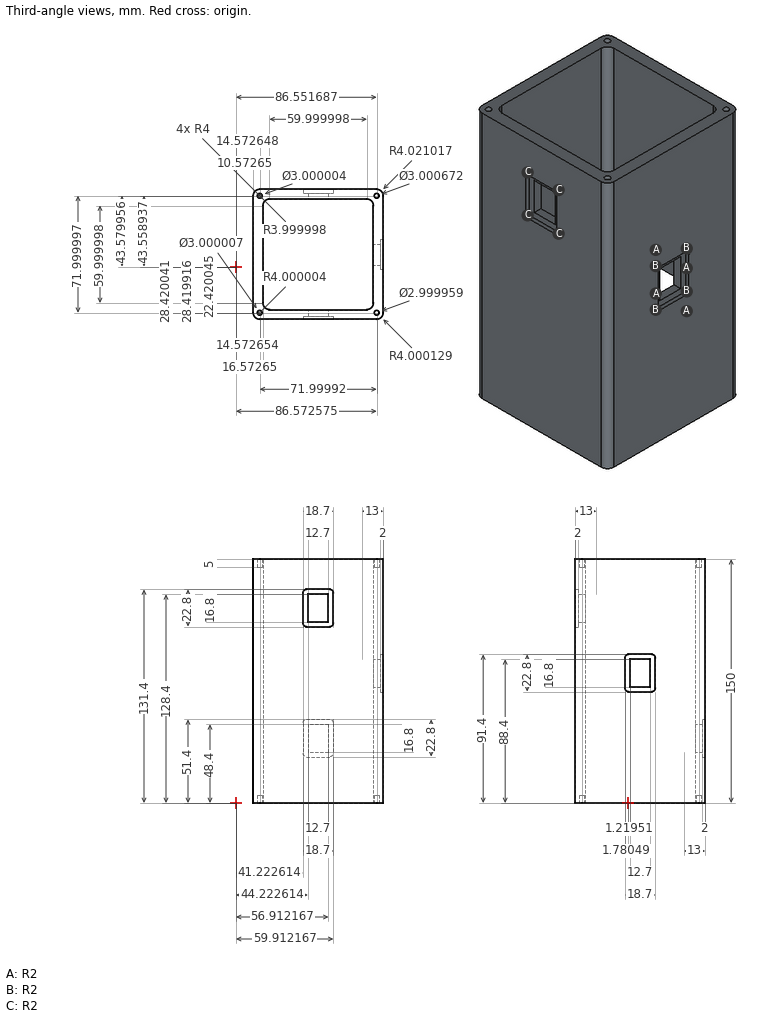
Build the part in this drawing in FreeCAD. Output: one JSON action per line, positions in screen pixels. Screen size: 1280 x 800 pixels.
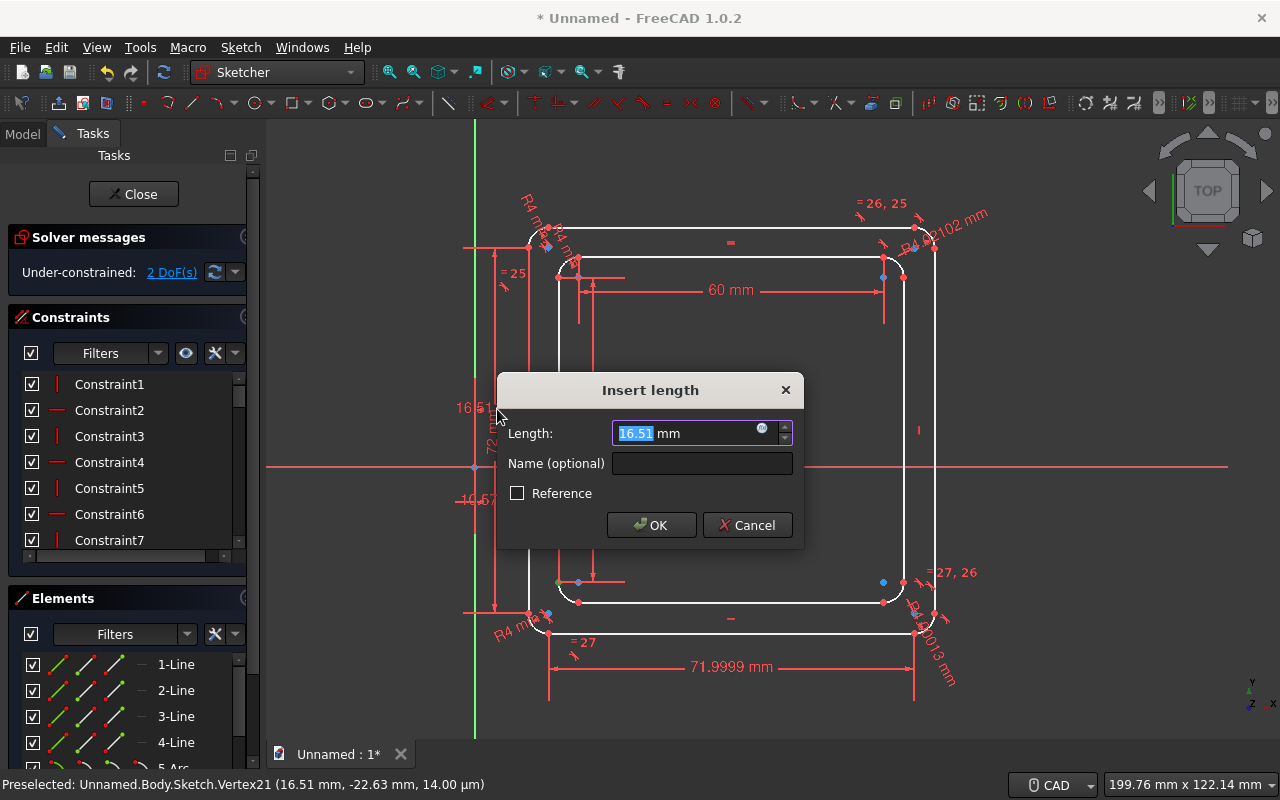
{"action": "type", "text": "16.57265"}
{"action": "key", "text": "Return"}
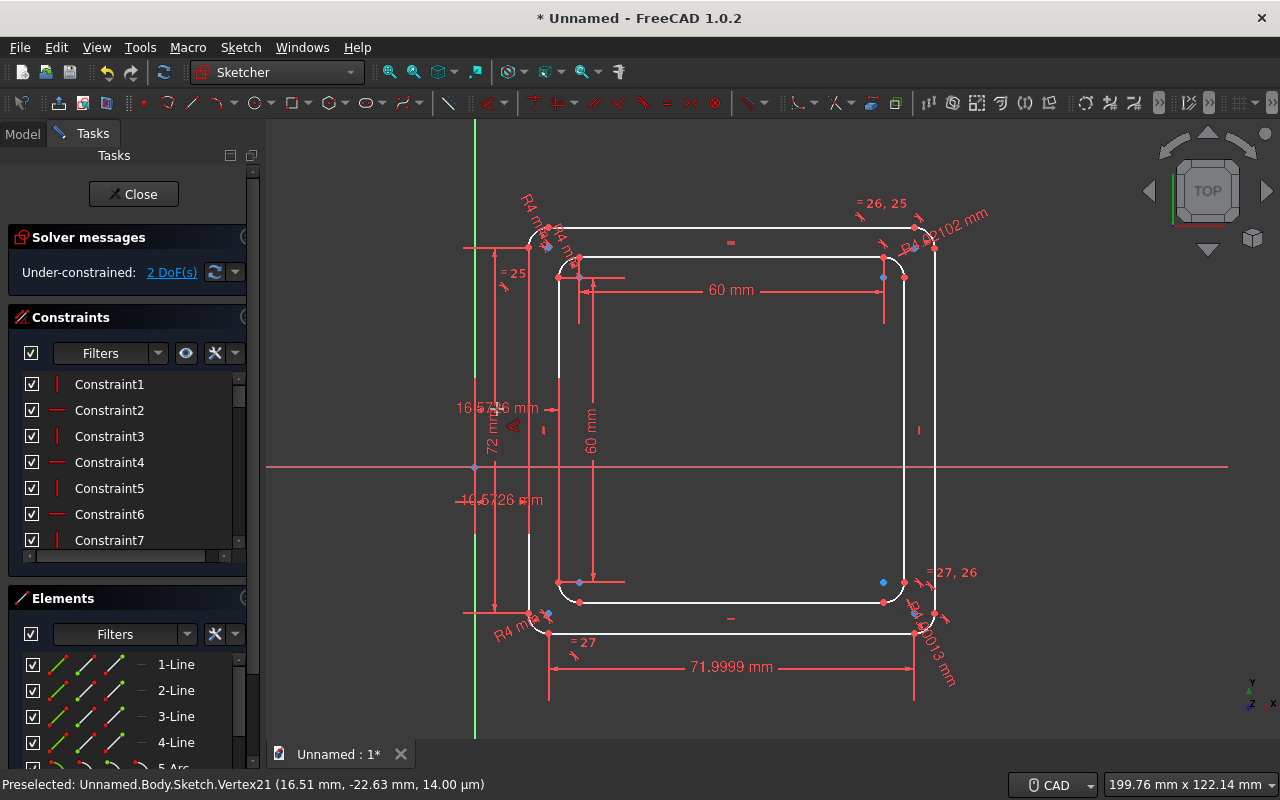
{"action": "left_click", "coordinate": [529, 248]}
{"action": "left_click", "coordinate": [441, 358]}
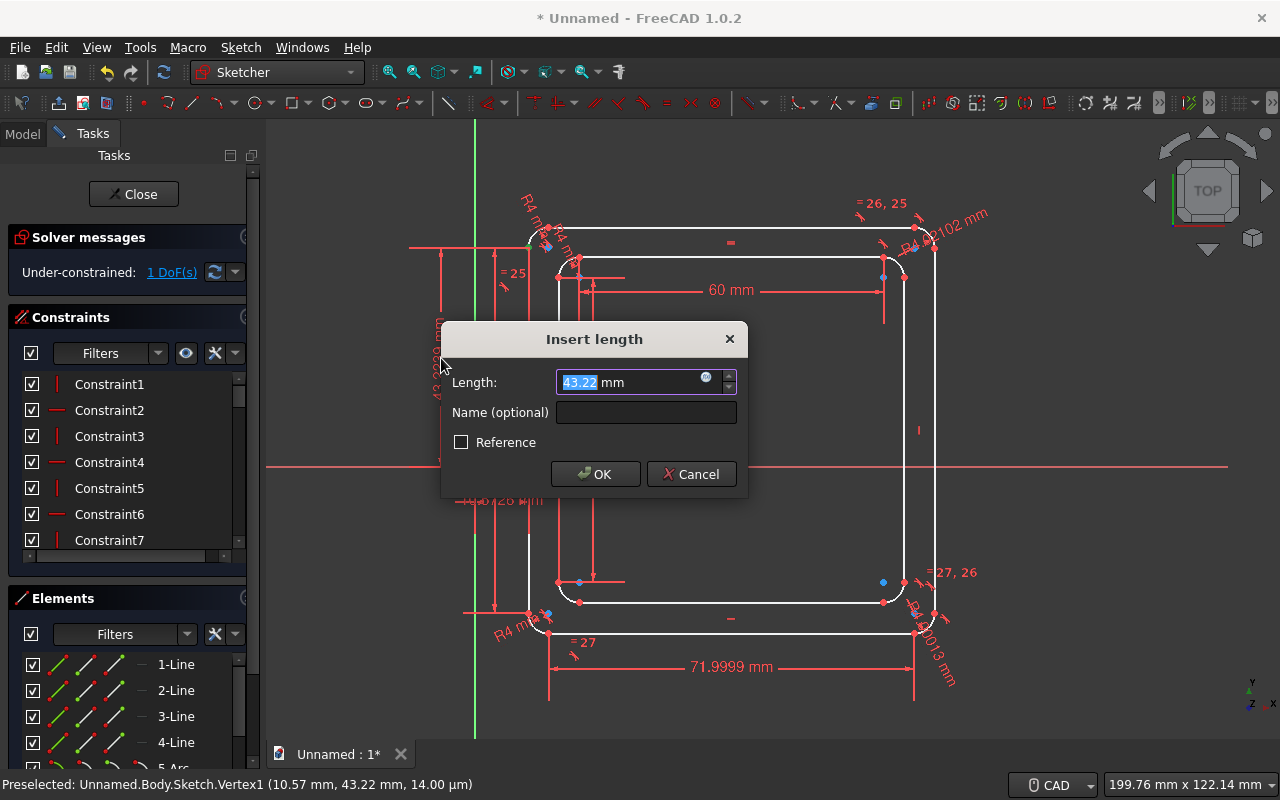
{"action": "type", "text": "43.579956"}
{"action": "key", "text": "Return"}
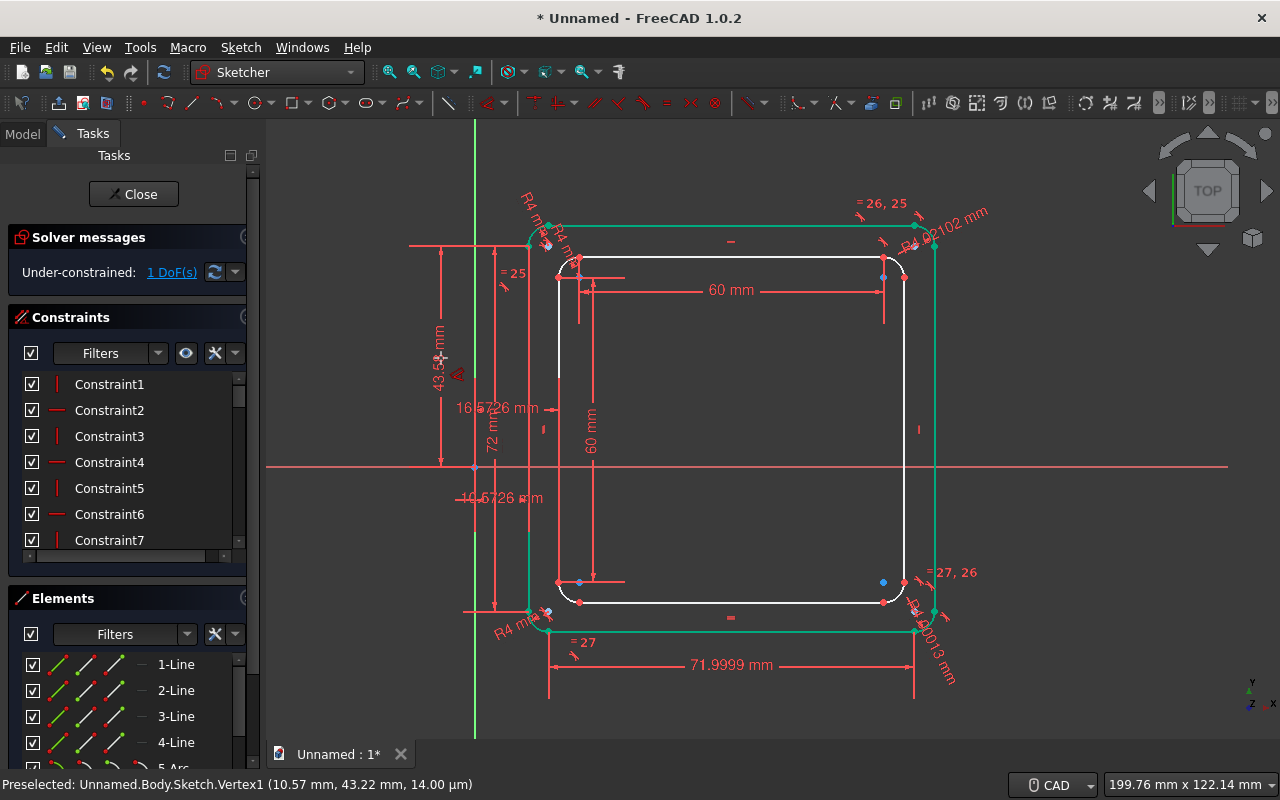
{"action": "left_click", "coordinate": [559, 582]}
{"action": "left_click", "coordinate": [441, 525]}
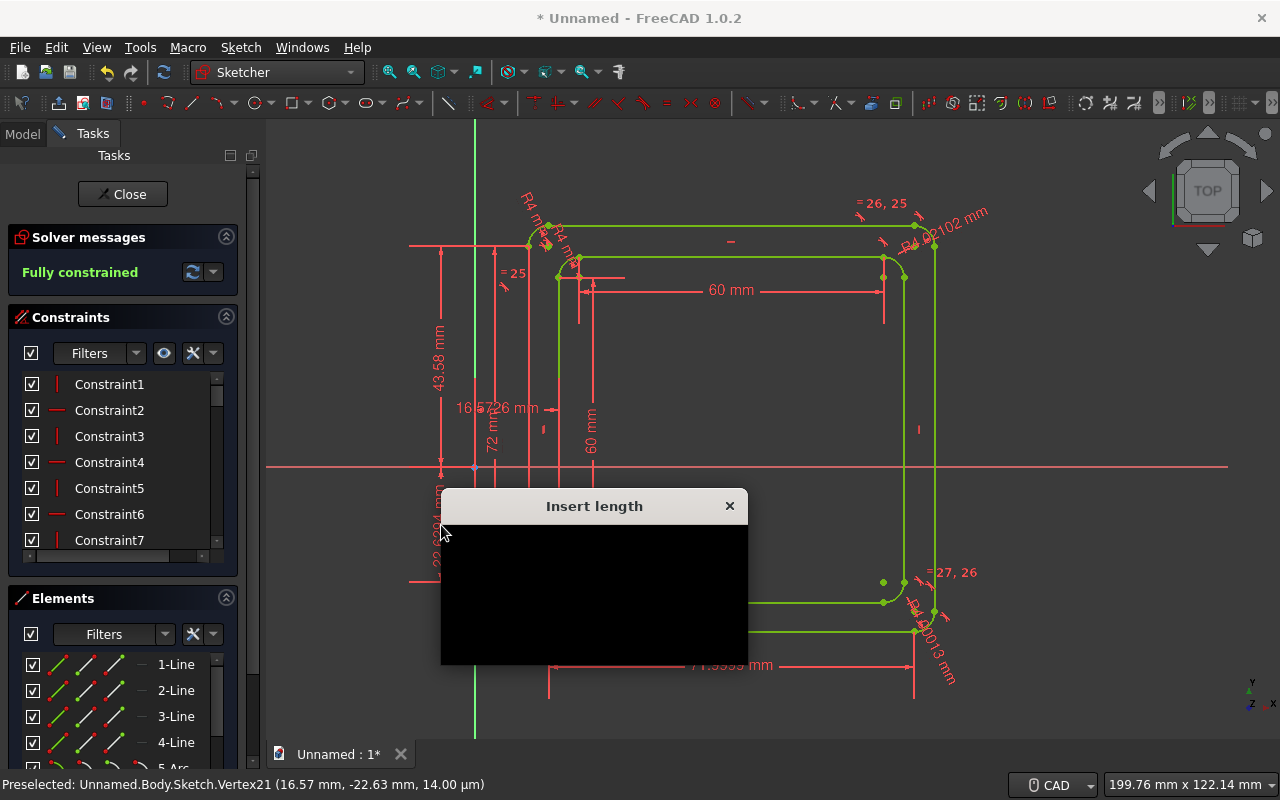
{"action": "type", "text": "22.420045"}
{"action": "key", "text": "Return"}
{"action": "key", "text": "Escape"}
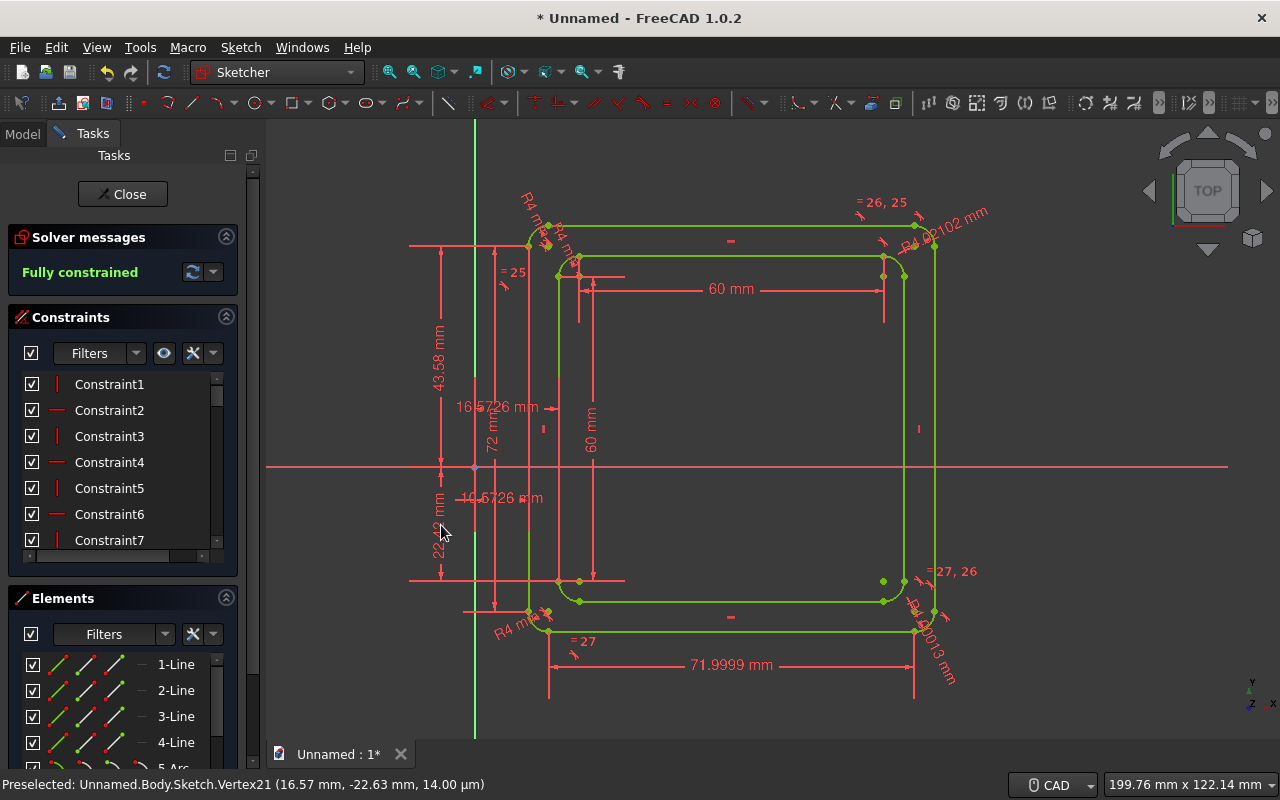
{"action": "left_click", "coordinate": [123, 194]}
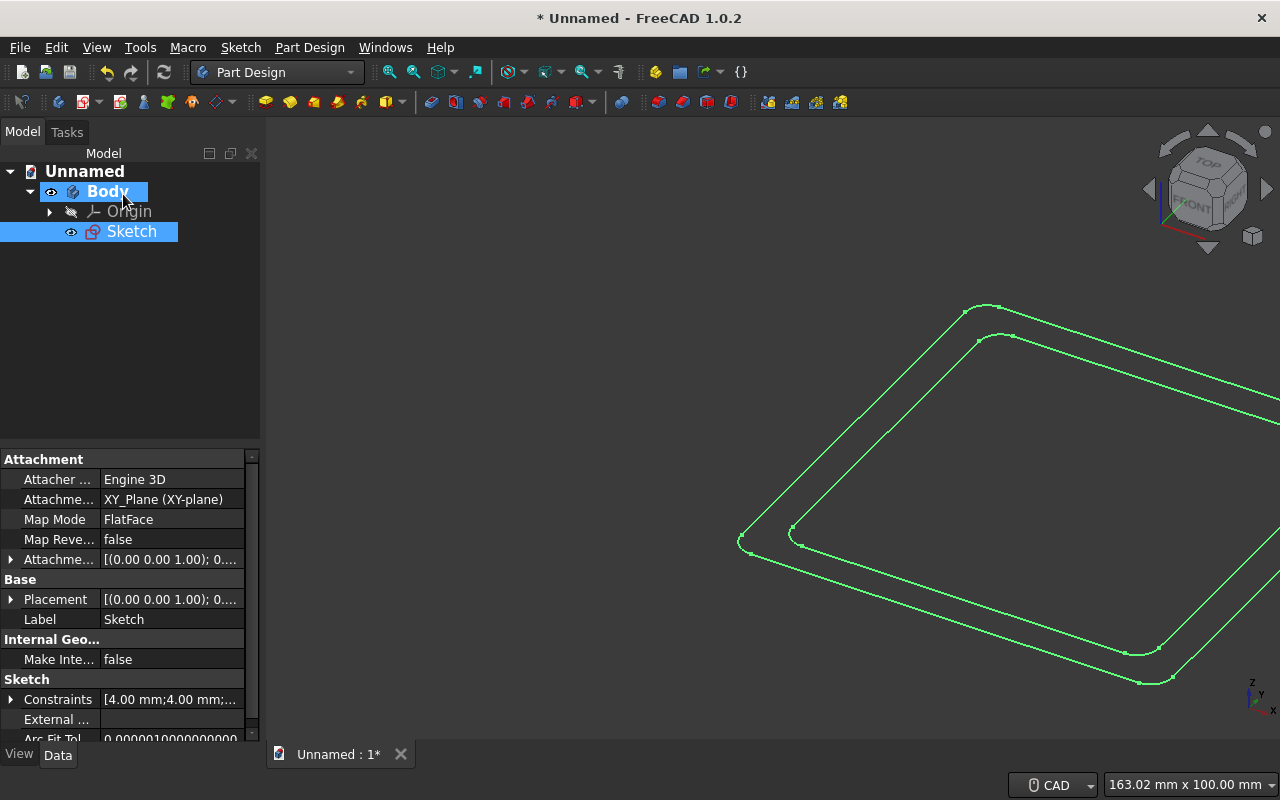
{"action": "left_click", "coordinate": [266, 102]}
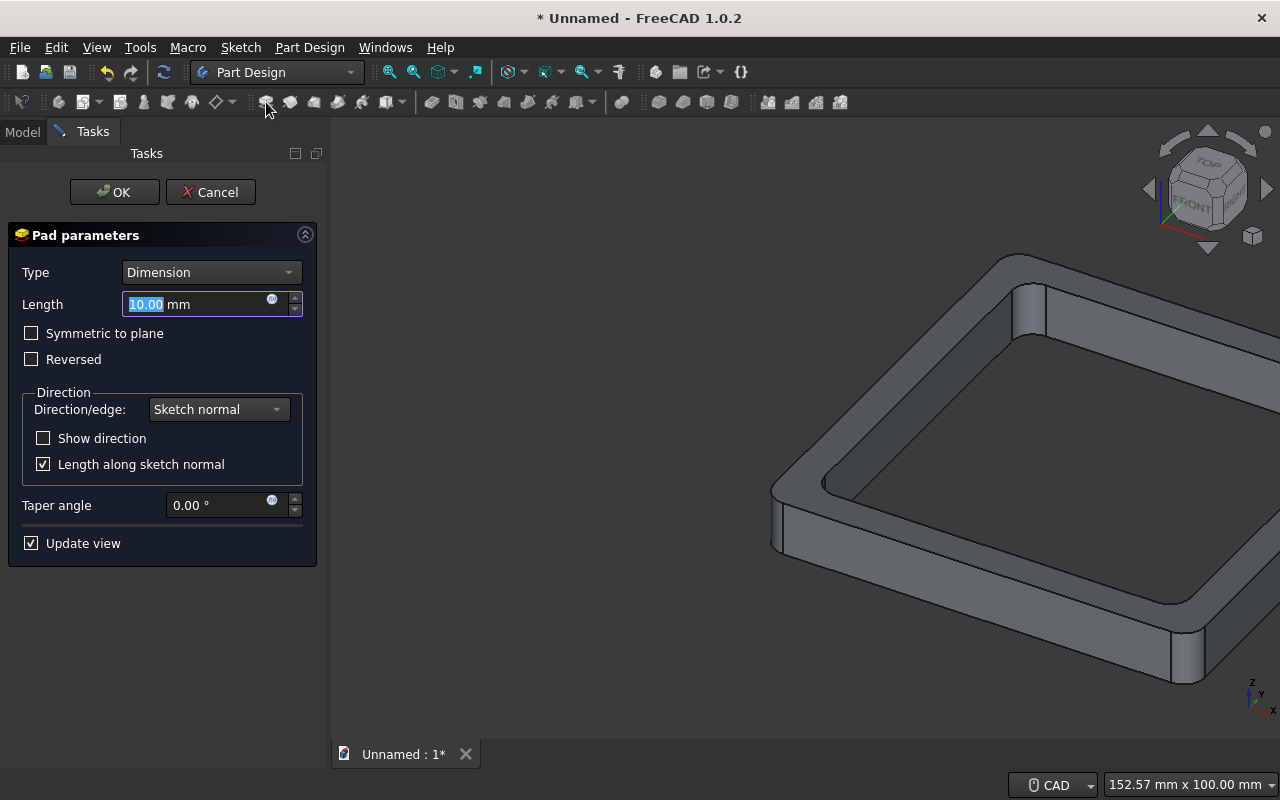
{"action": "type", "text": "150"}
{"action": "key", "text": "Tab"}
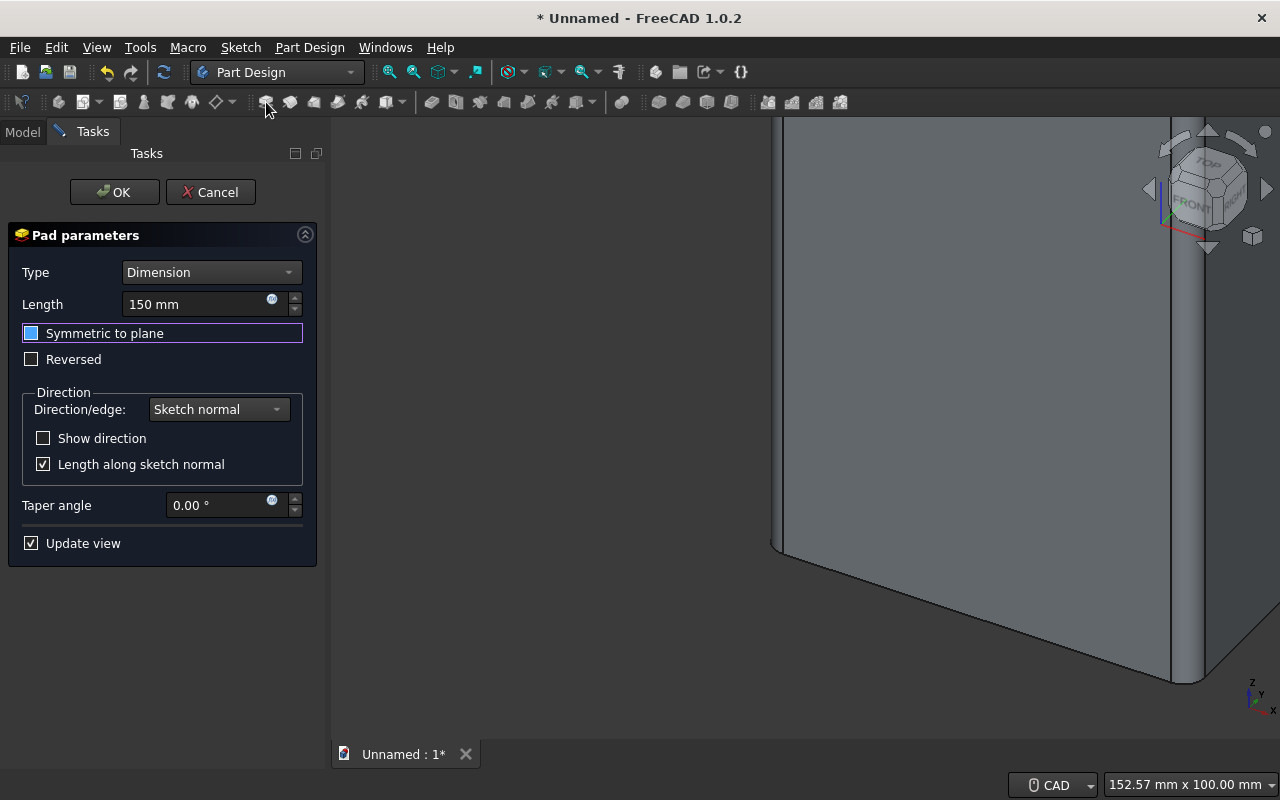
{"action": "left_click", "coordinate": [115, 192]}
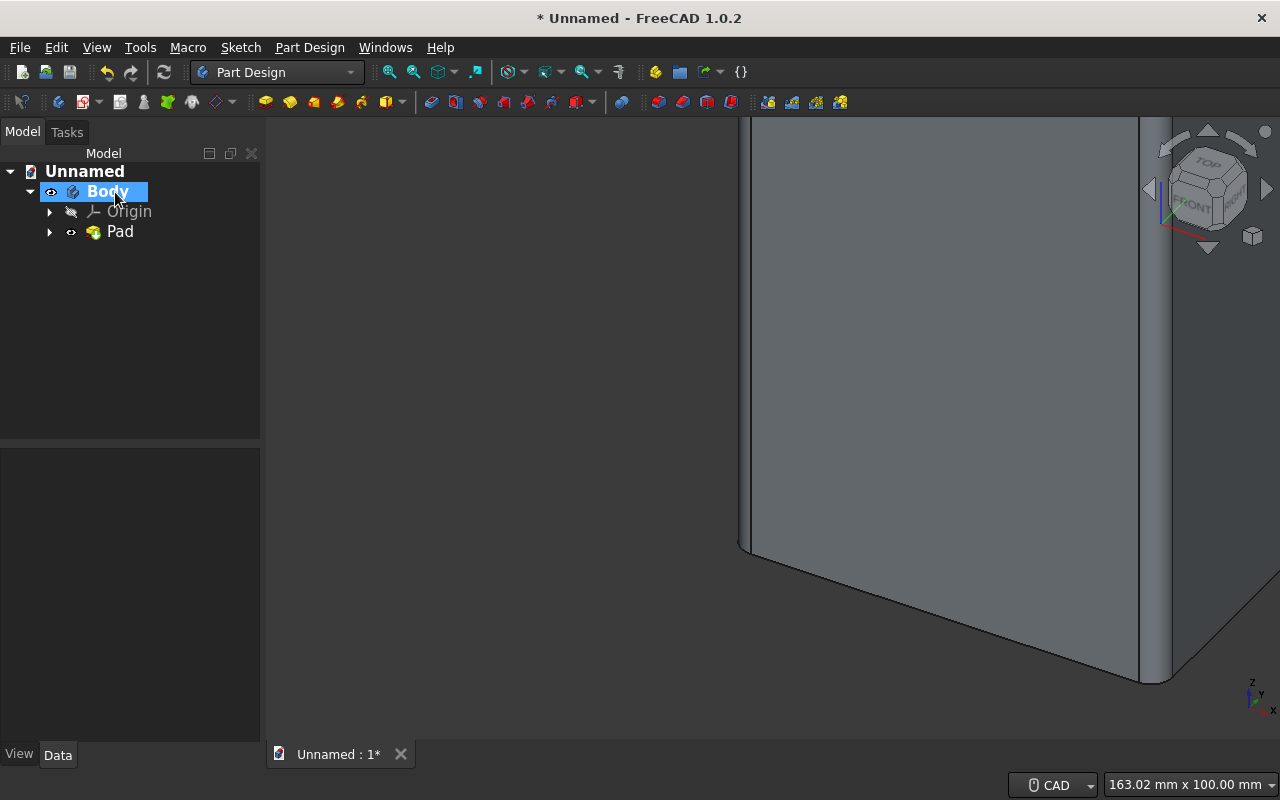
{"action": "left_click", "coordinate": [390, 72]}